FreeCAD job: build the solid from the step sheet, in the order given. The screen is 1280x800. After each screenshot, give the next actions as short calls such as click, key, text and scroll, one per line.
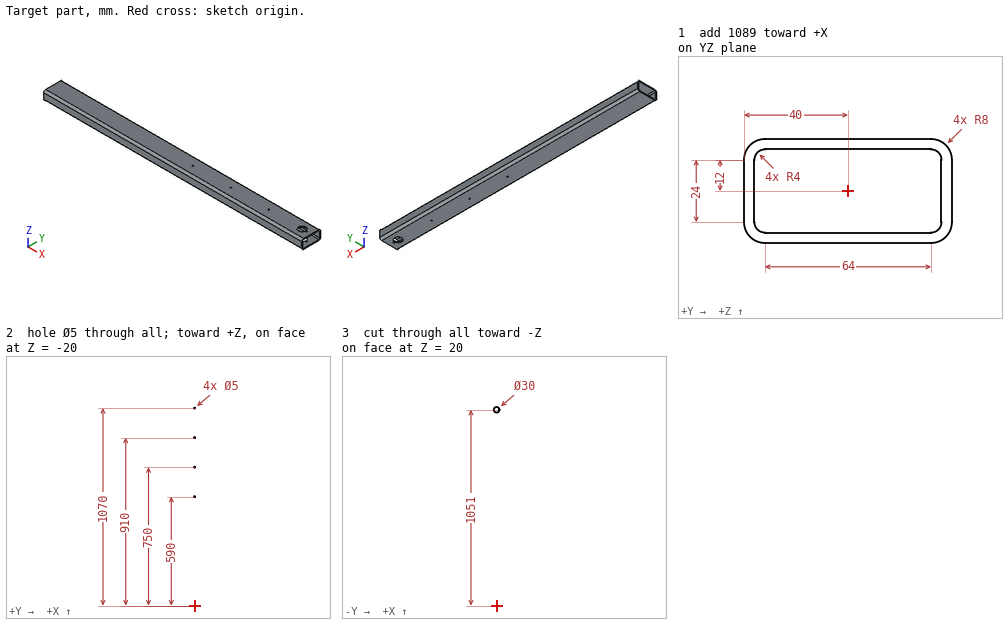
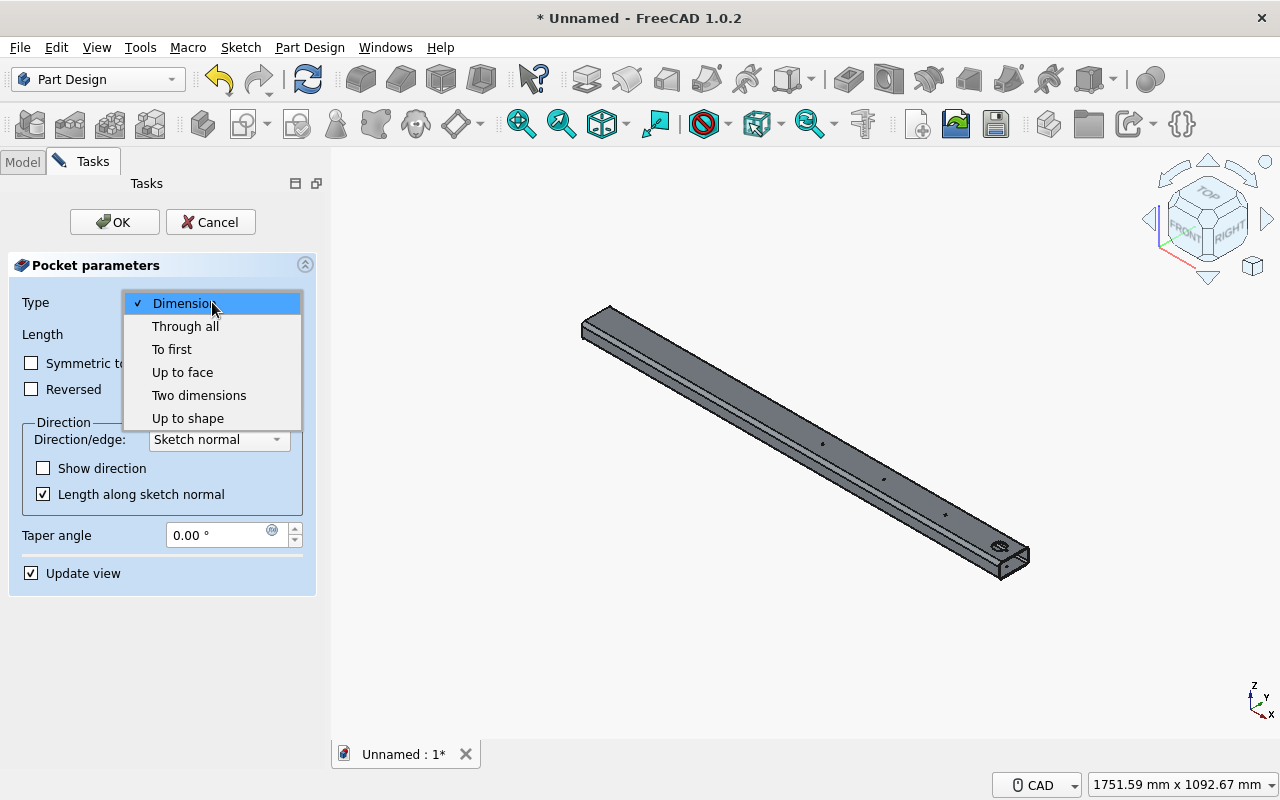
click(212, 326)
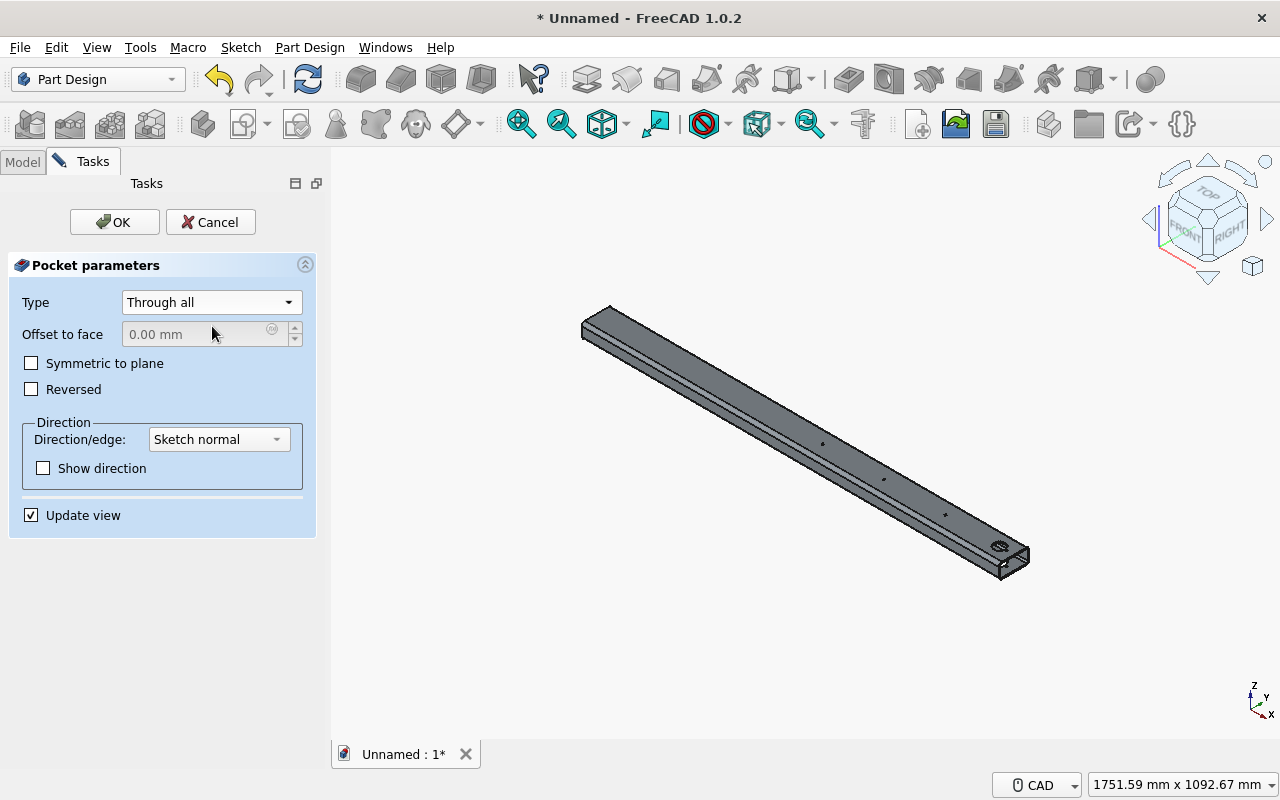
click(115, 222)